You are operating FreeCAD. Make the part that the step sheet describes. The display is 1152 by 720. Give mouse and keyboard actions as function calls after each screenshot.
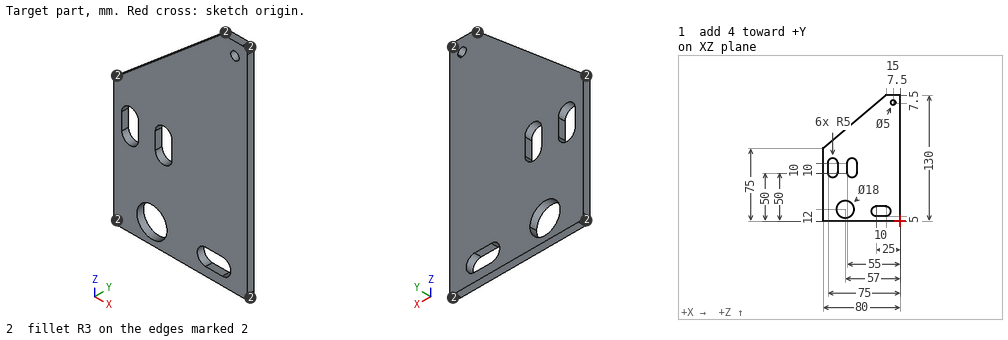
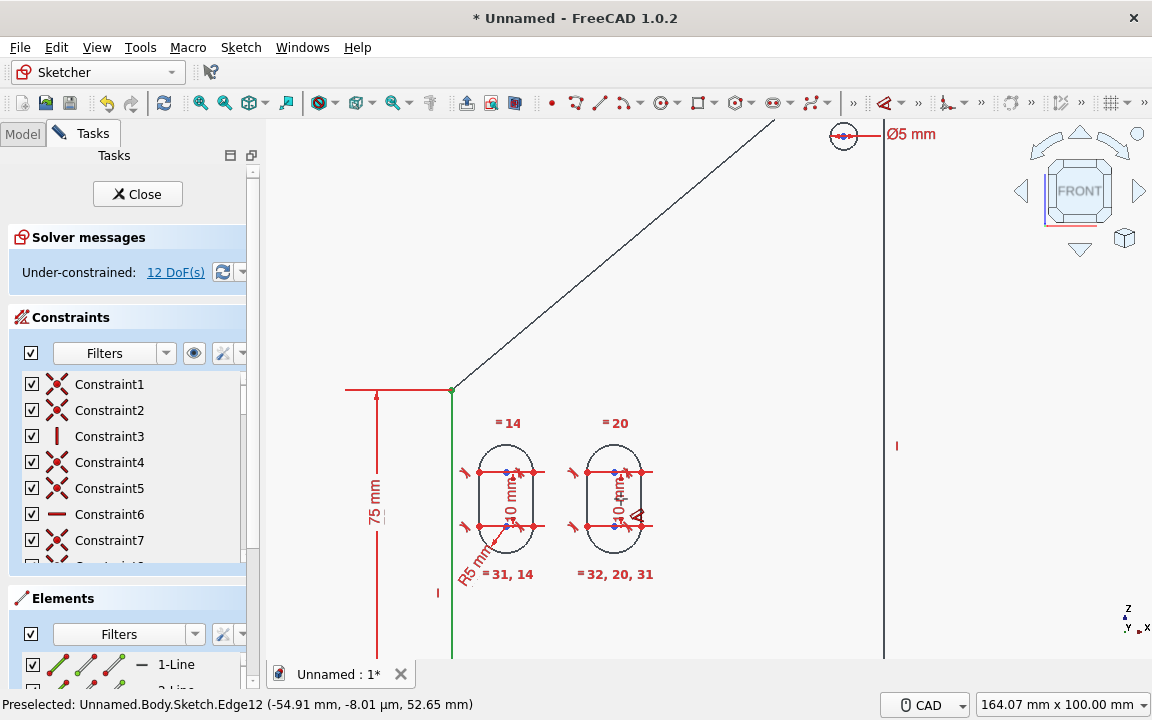
scroll(618, 344, down, 4)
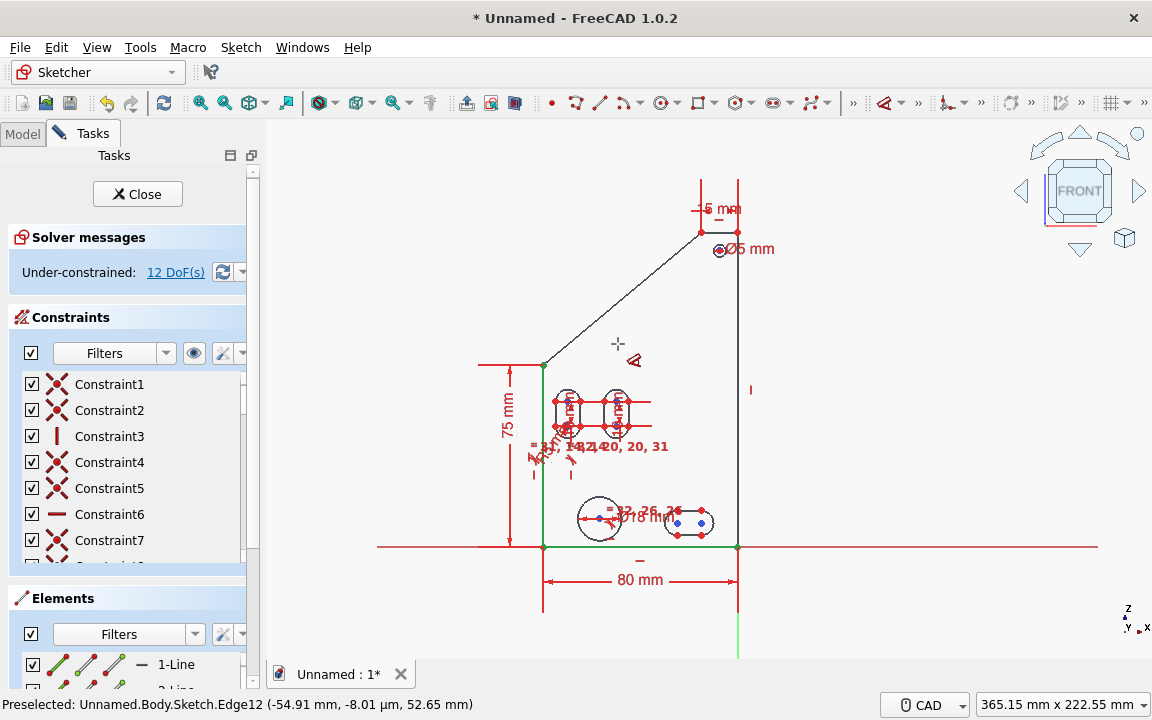
scroll(684, 511, up, 4)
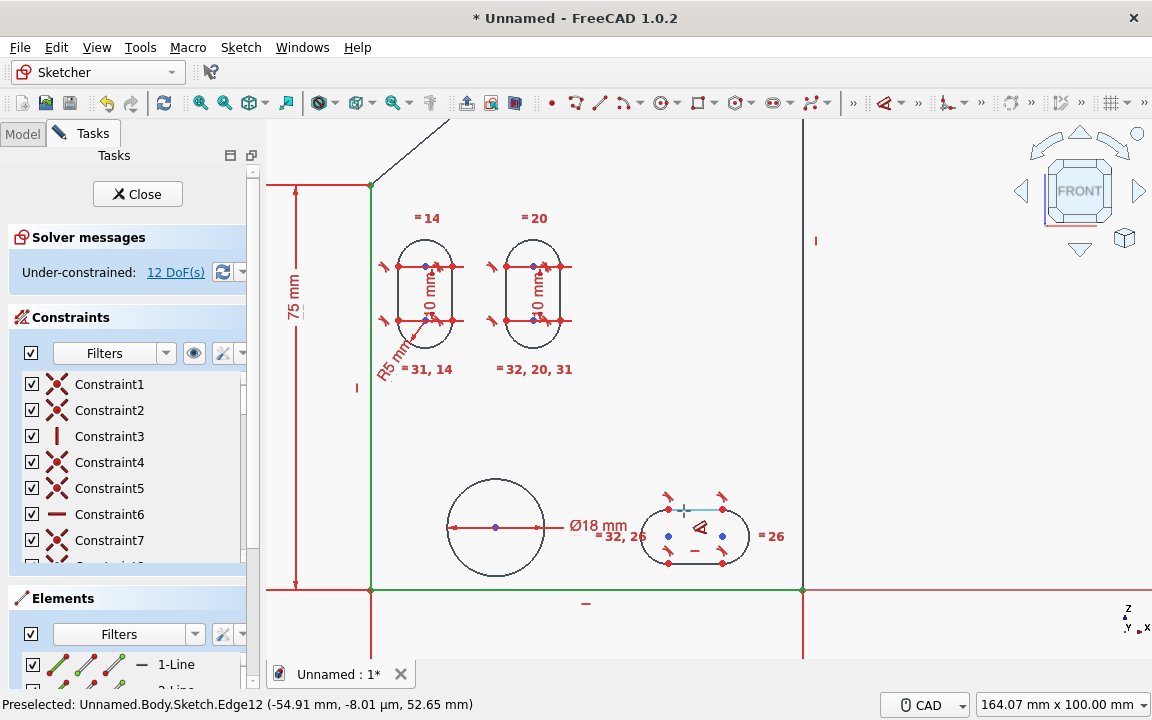
click(684, 510)
click(695, 544)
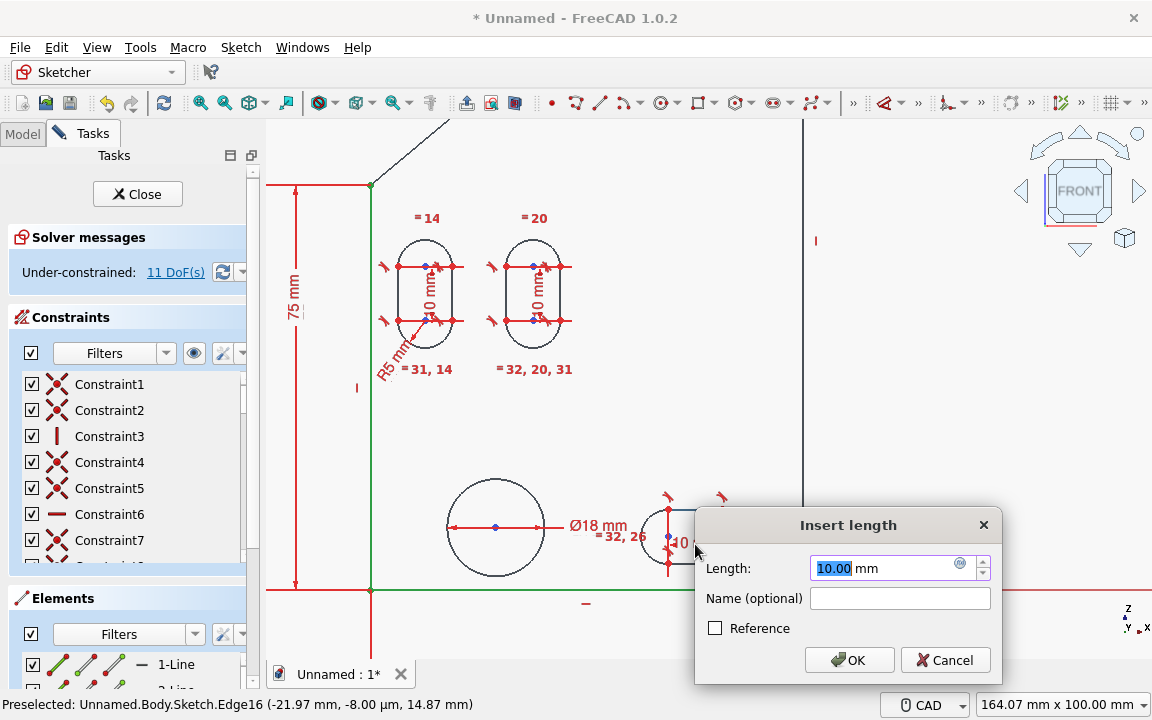
text(10)
key(Return)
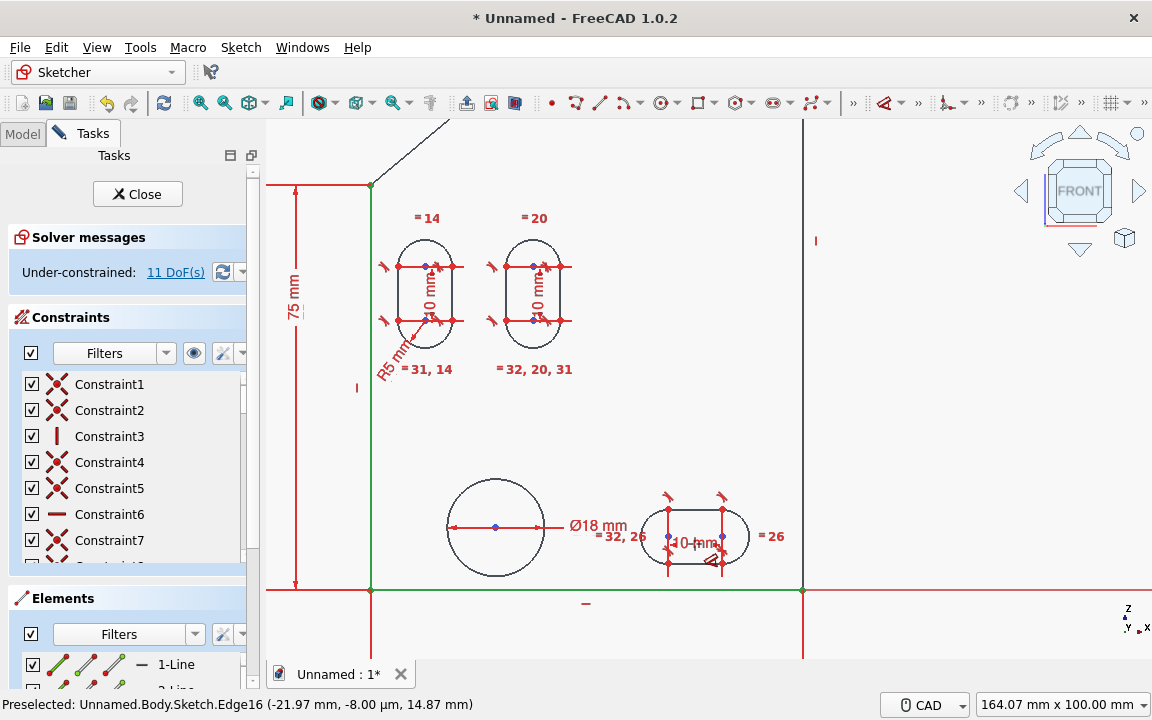
scroll(668, 564, up, 2)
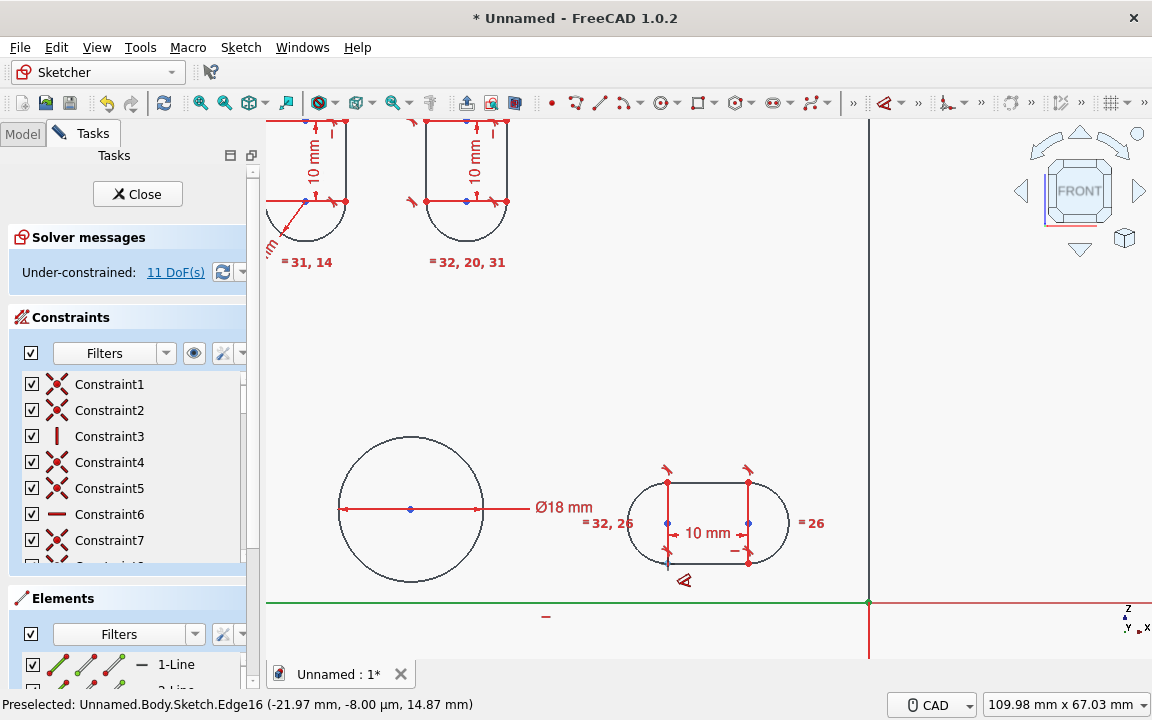
click(668, 564)
click(903, 583)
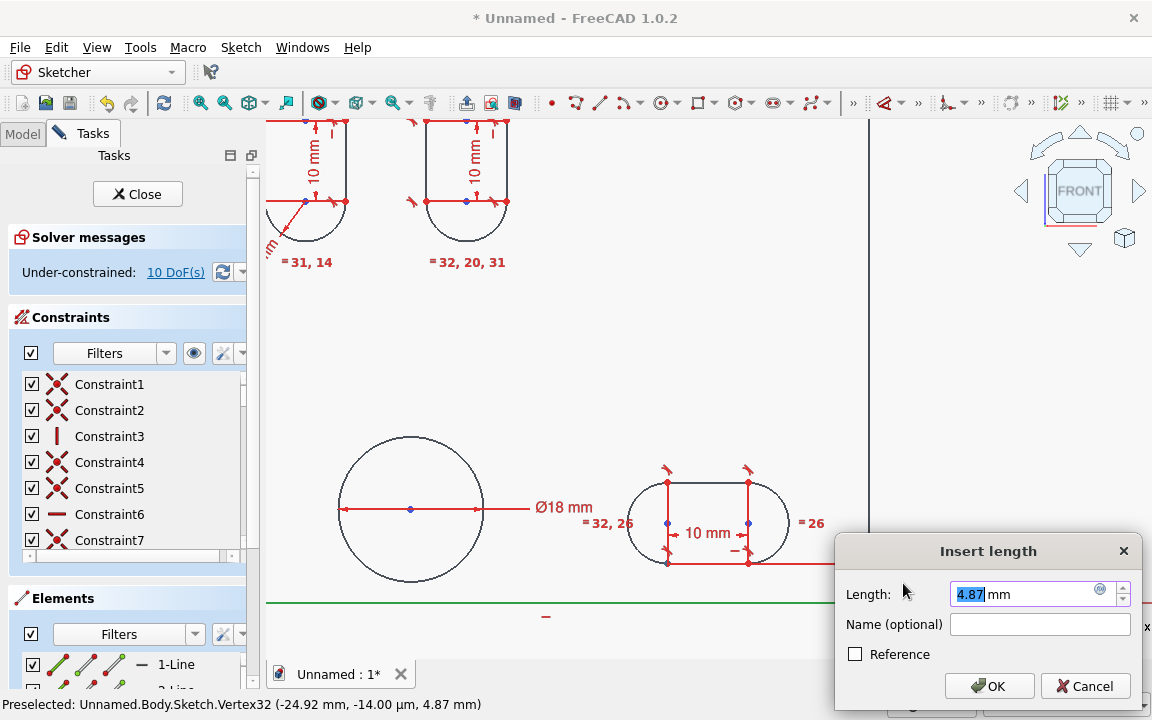
text(5)
key(Return)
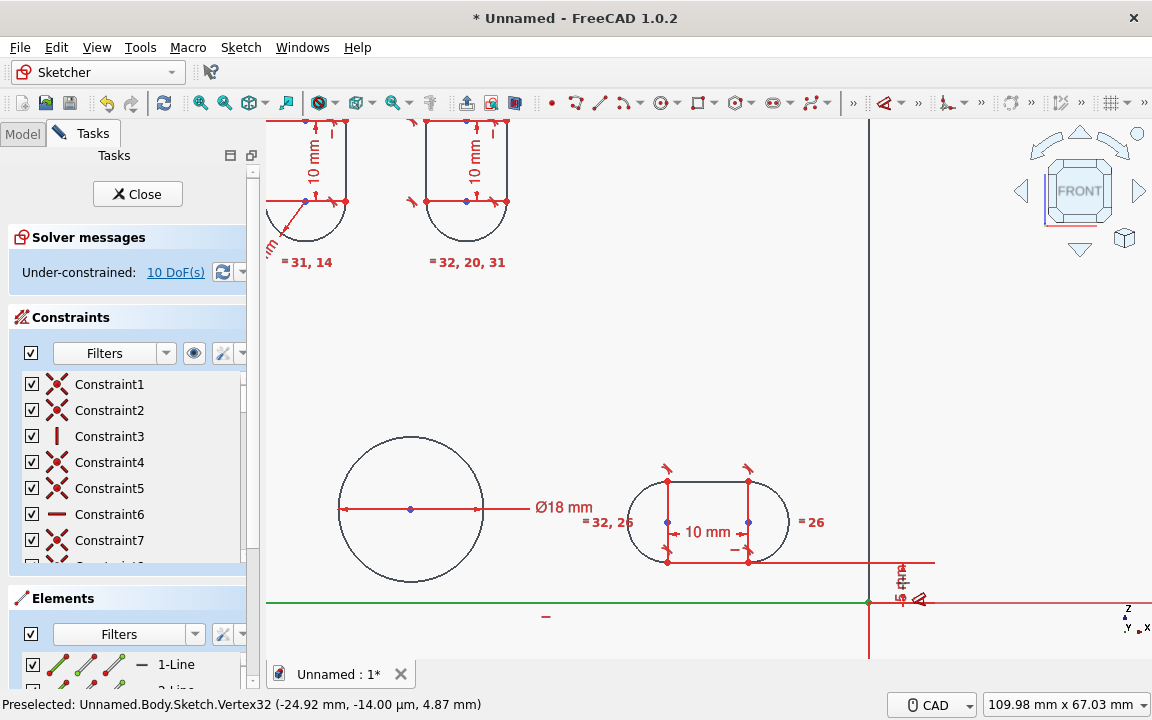
click(411, 509)
click(640, 475)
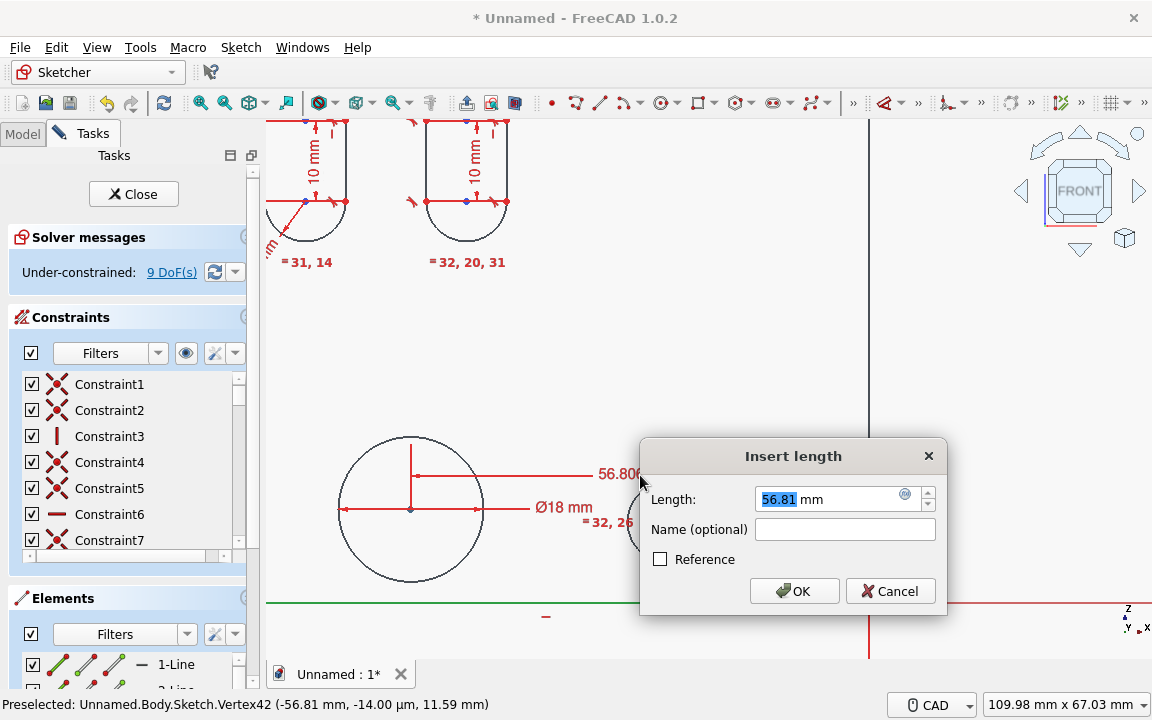
text(57)
key(Return)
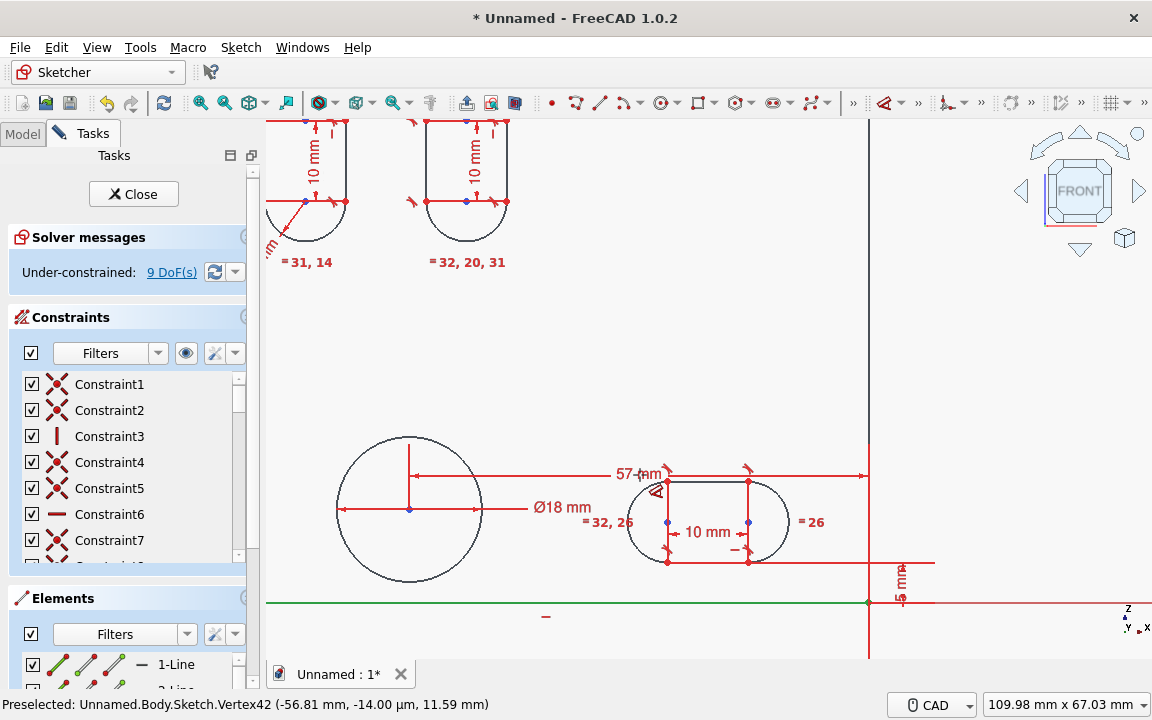
click(409, 509)
click(903, 556)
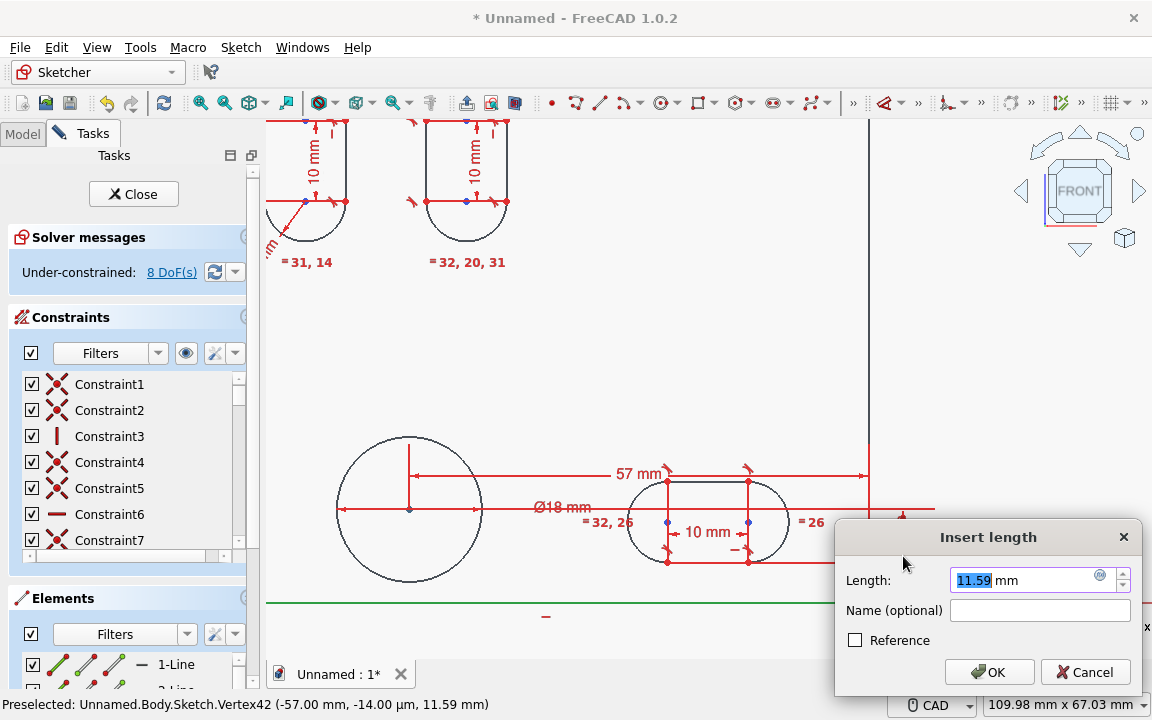
text(12)
key(Return)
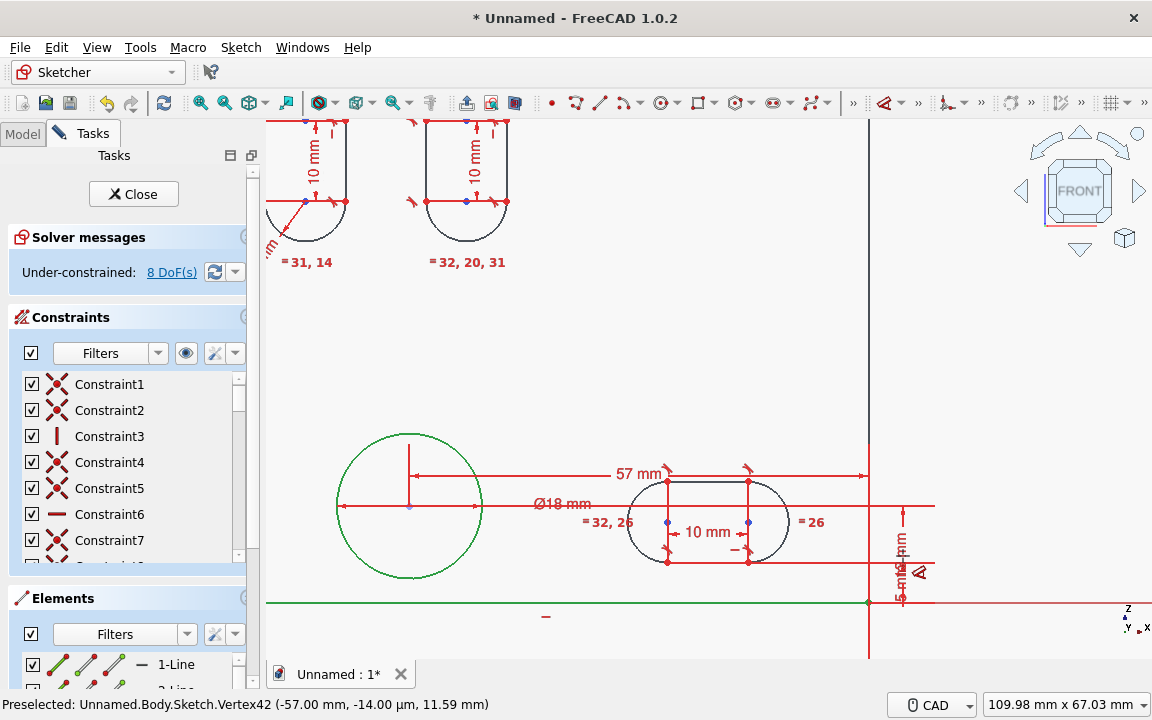
click(869, 290)
click(903, 375)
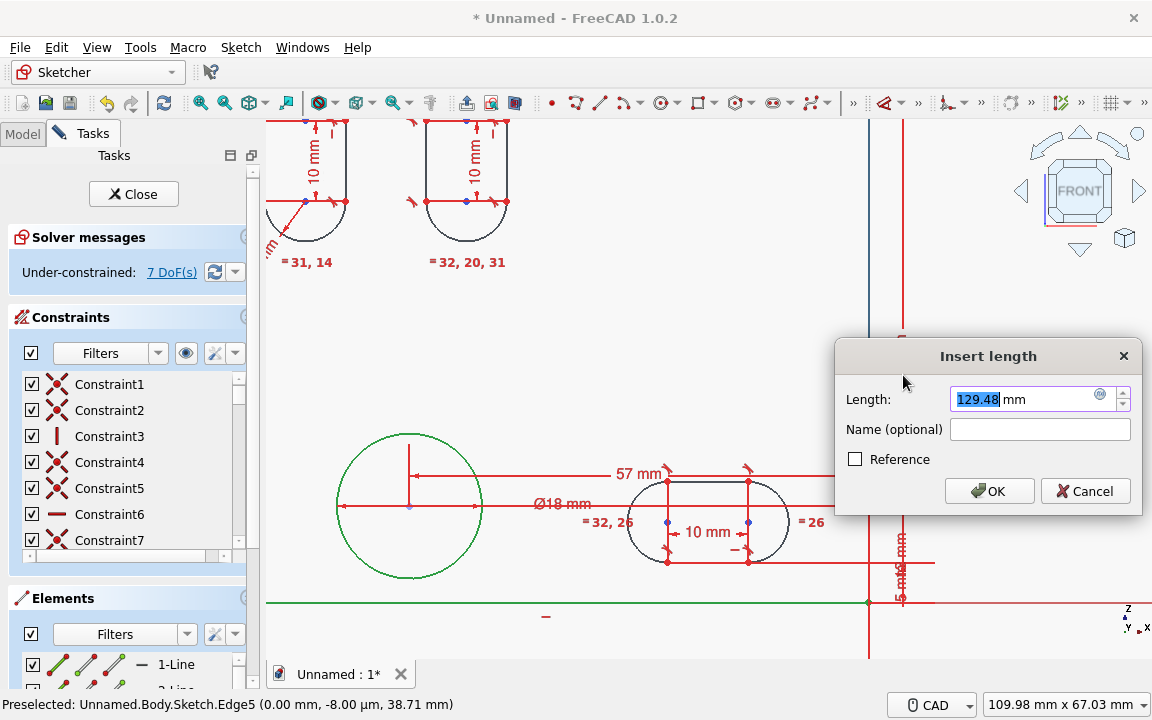
text(130)
key(Return)